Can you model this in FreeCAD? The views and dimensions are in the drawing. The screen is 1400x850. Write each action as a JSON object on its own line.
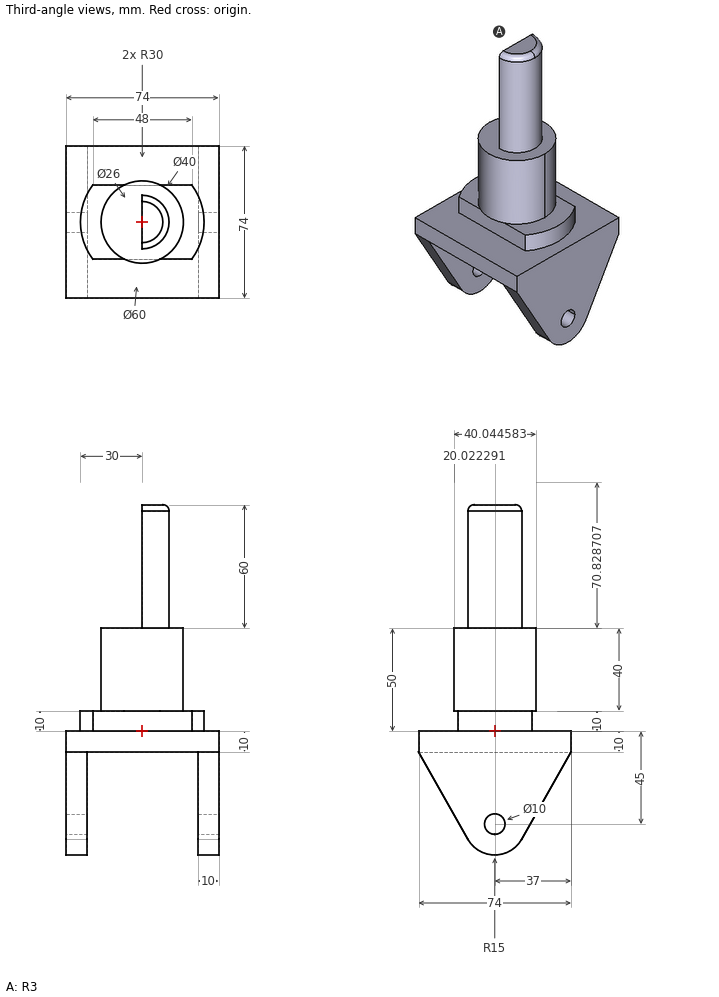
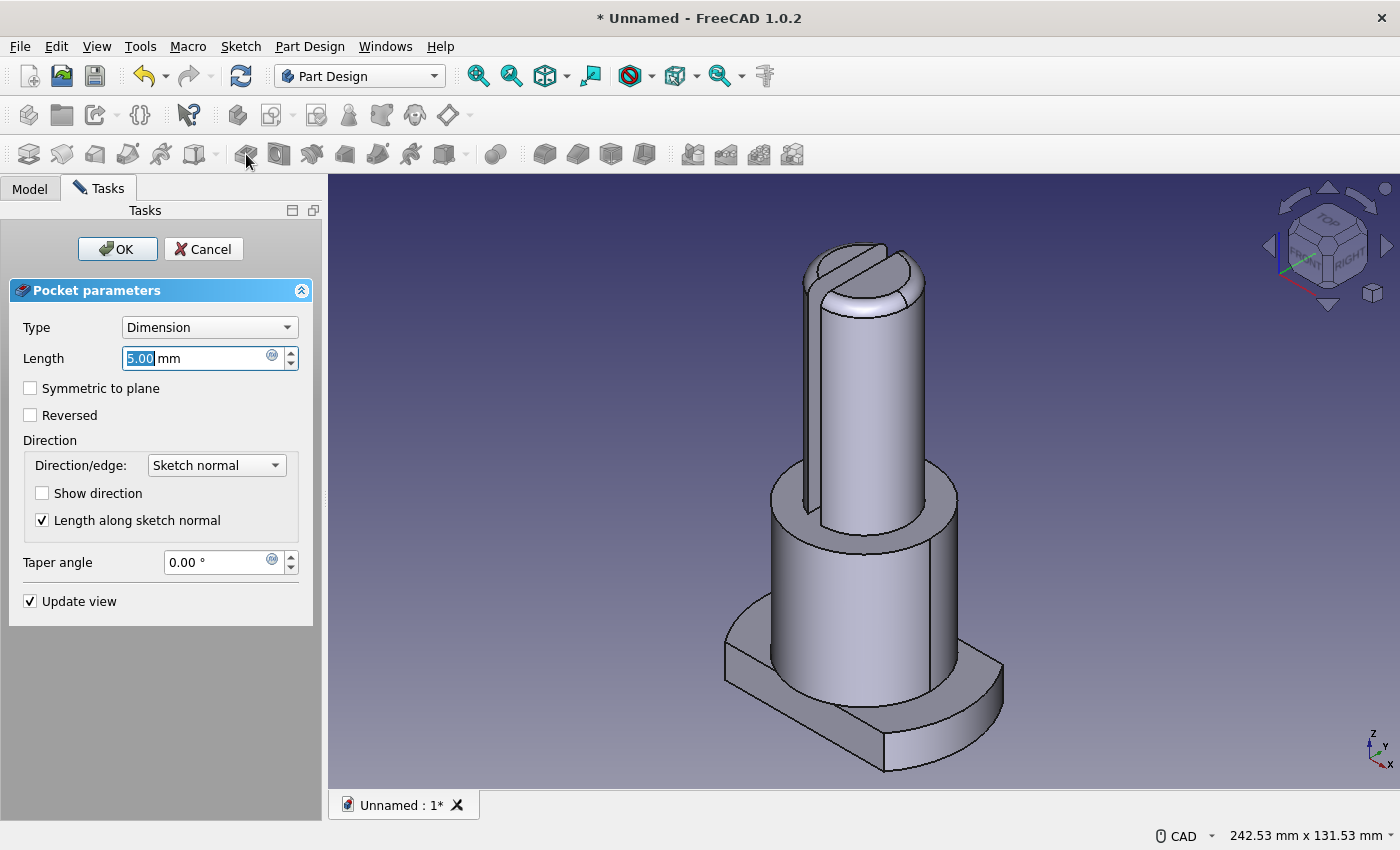
{"action": "type", "text": "30"}
{"action": "key", "text": "Tab"}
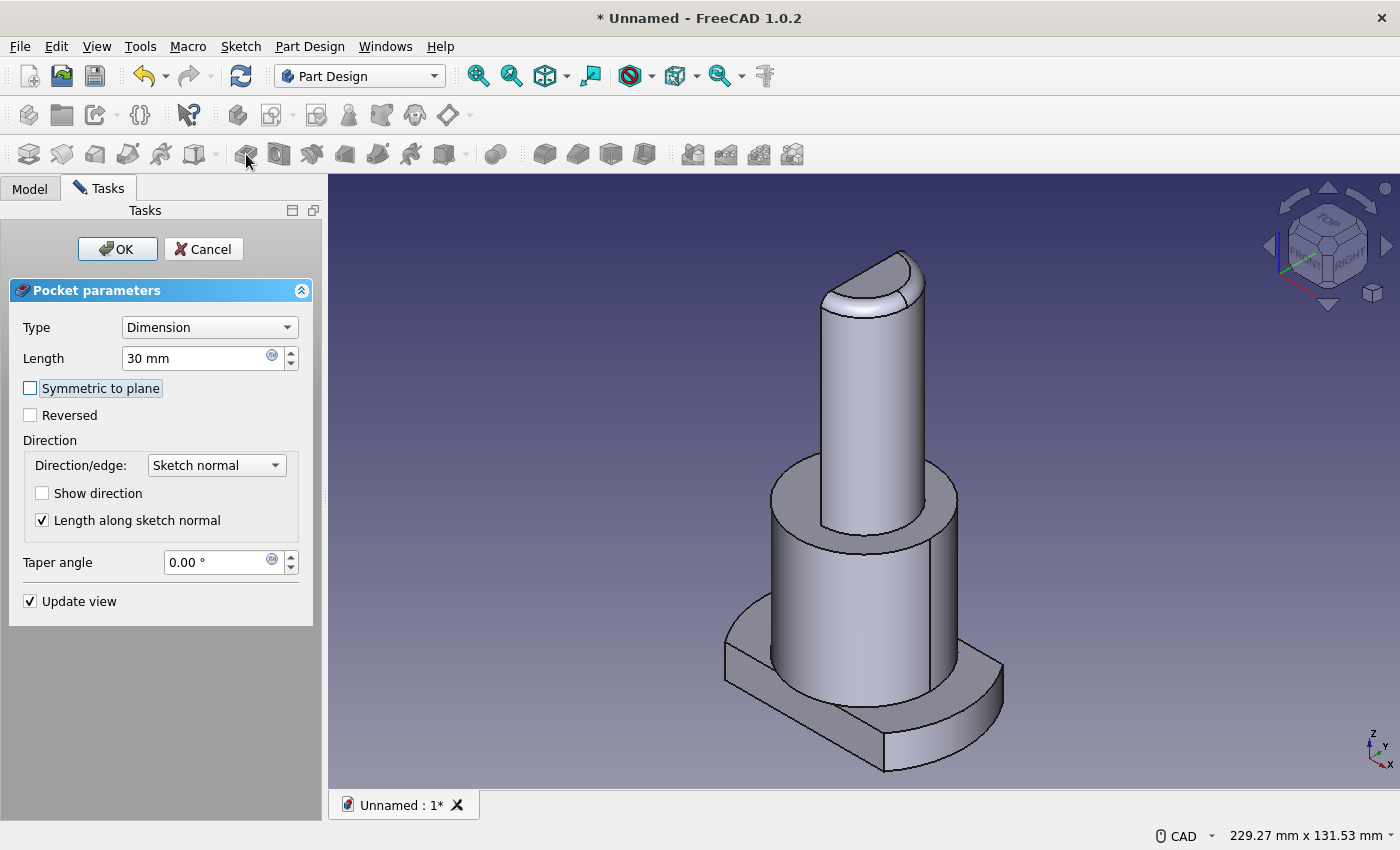
{"action": "left_click", "coordinate": [118, 249]}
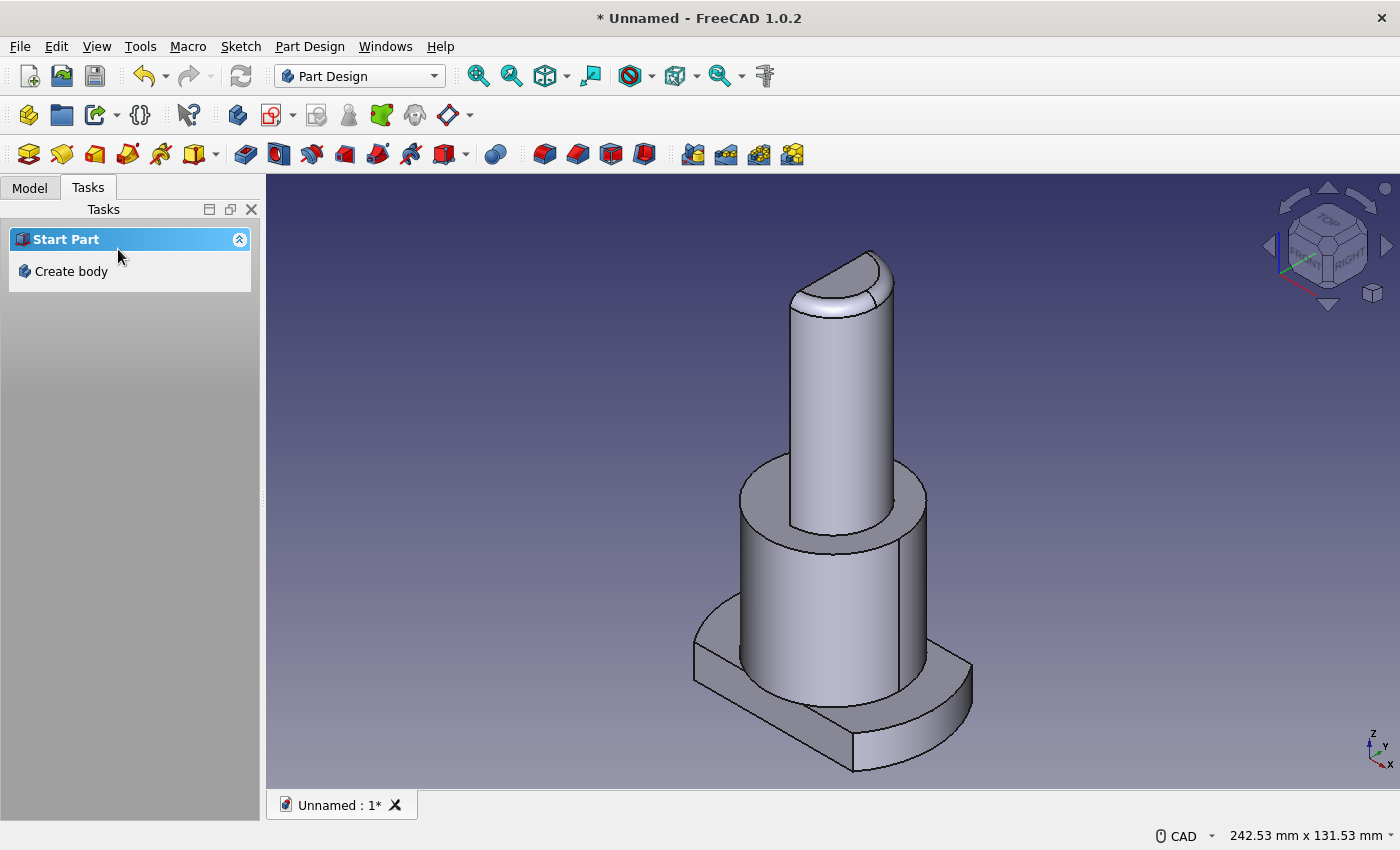
{"action": "key", "text": "5"}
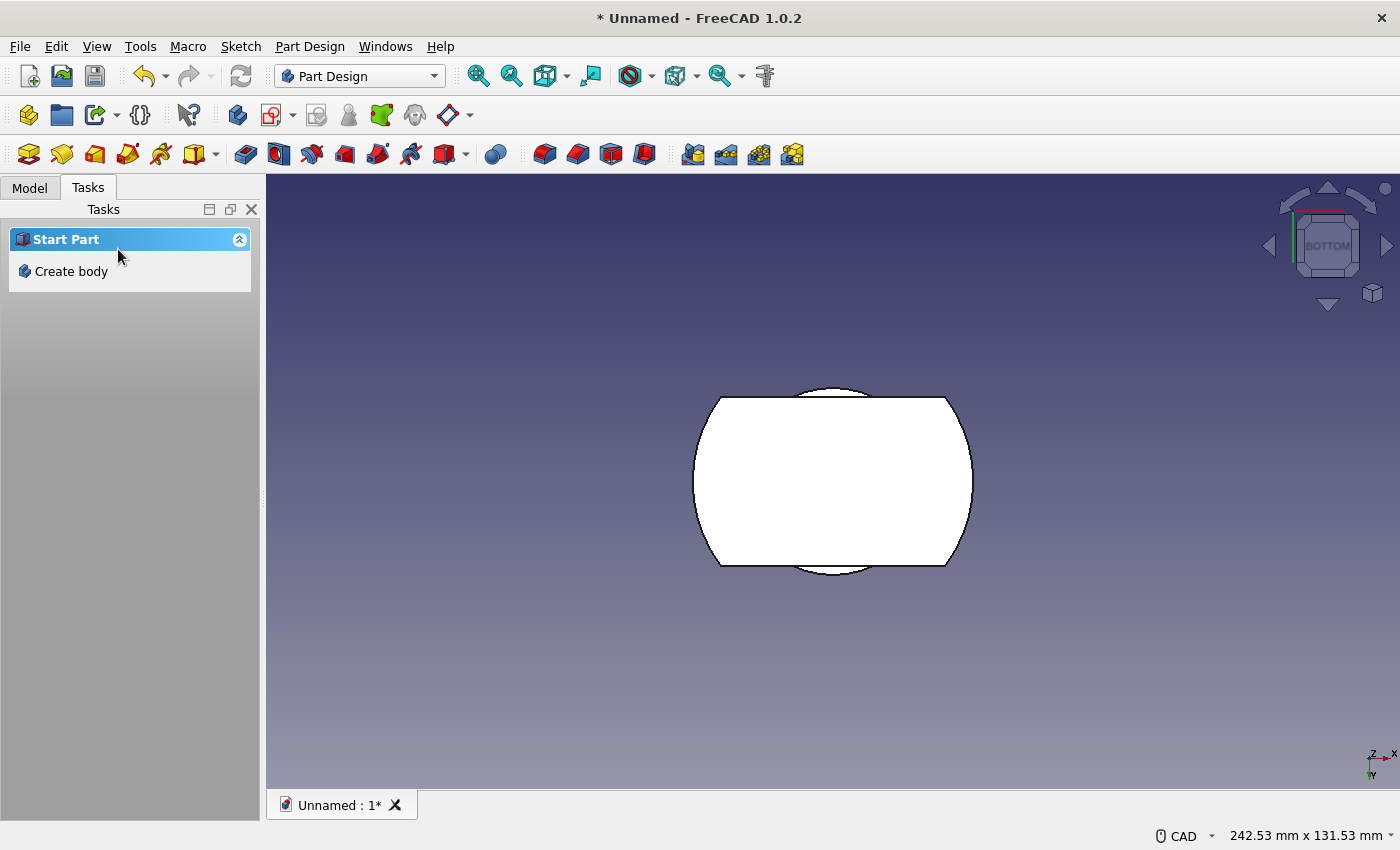
{"action": "left_click", "coordinate": [479, 76]}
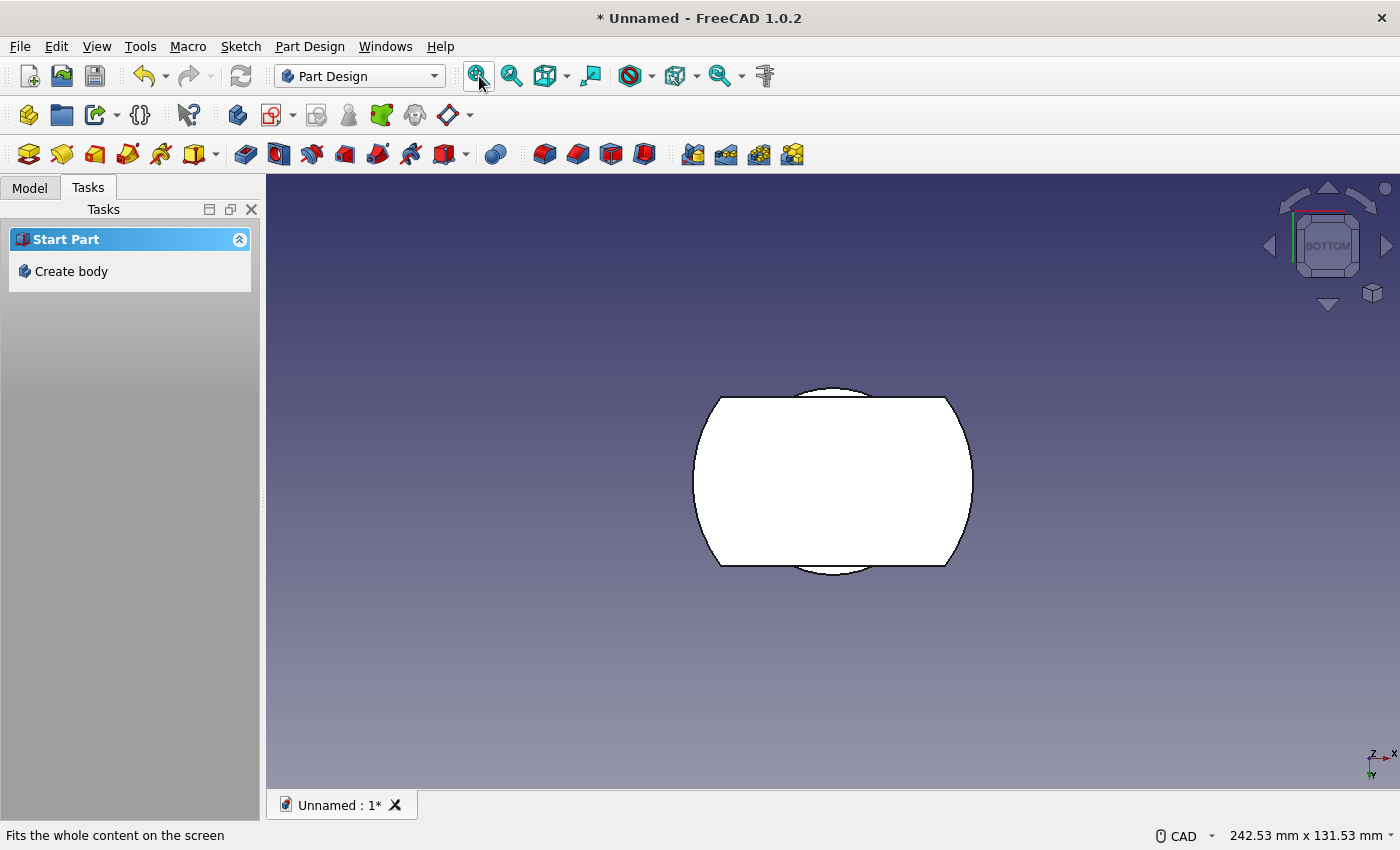
{"action": "left_click", "coordinate": [873, 480]}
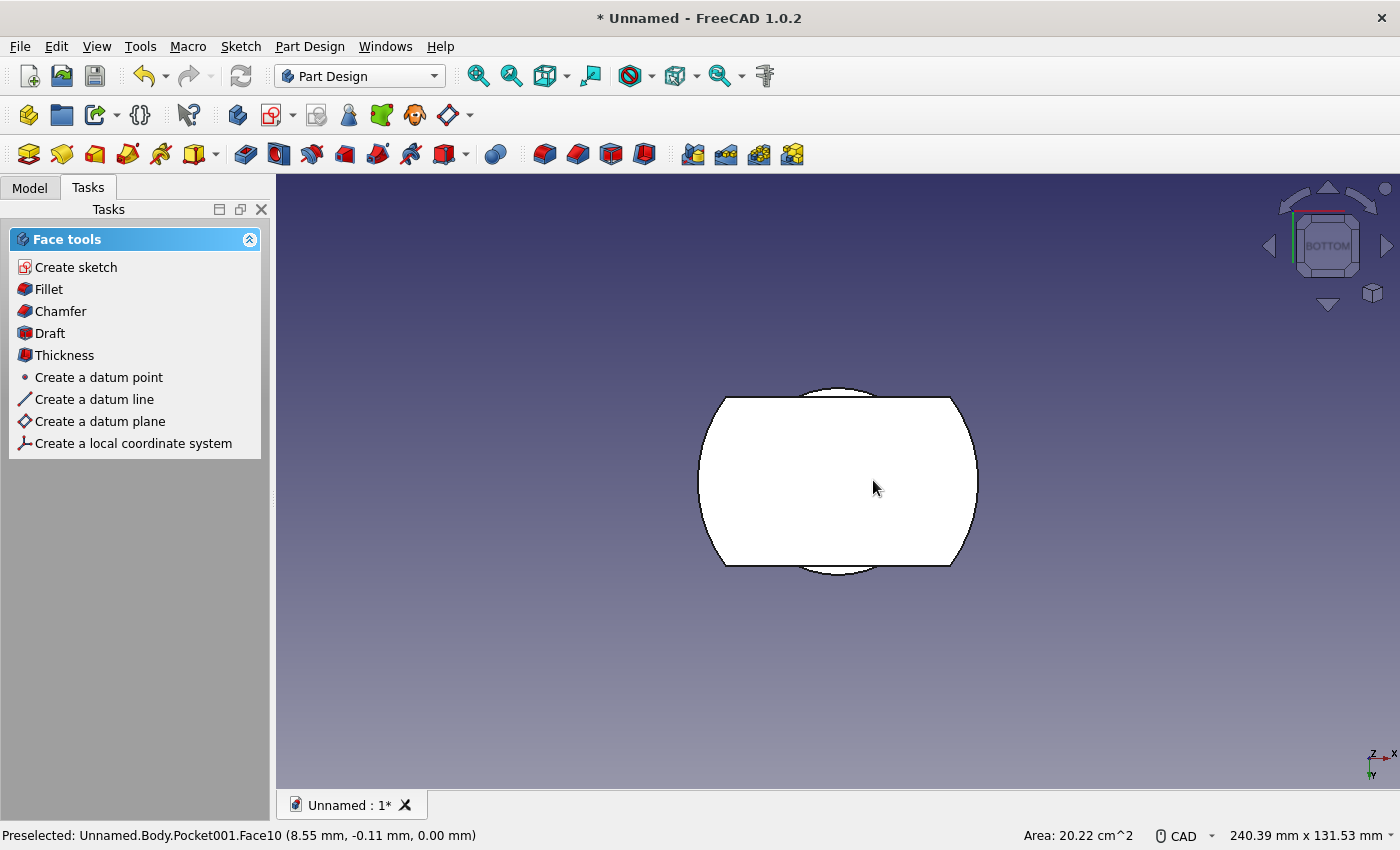
{"action": "left_click", "coordinate": [270, 116]}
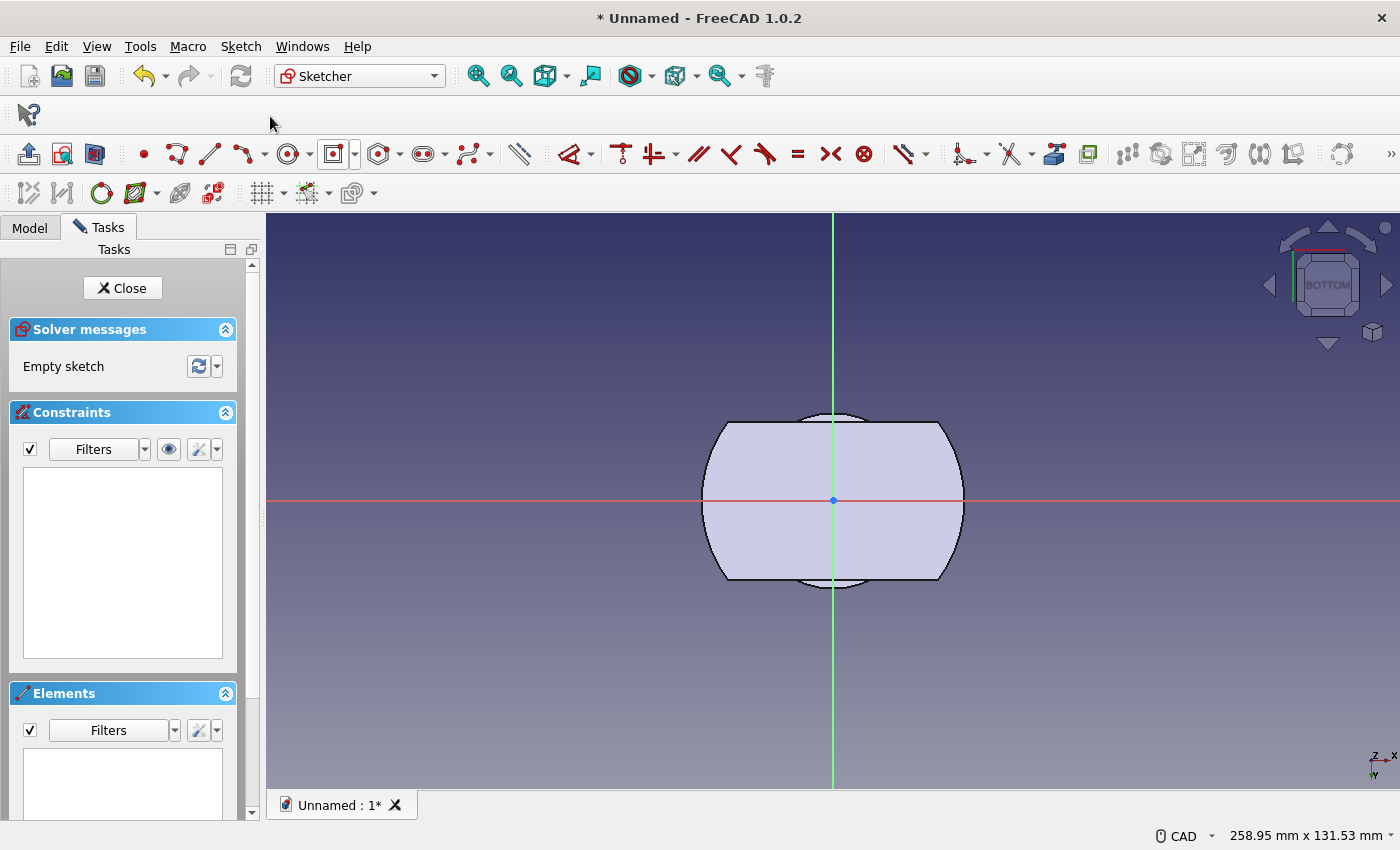
{"action": "key", "text": "g v"}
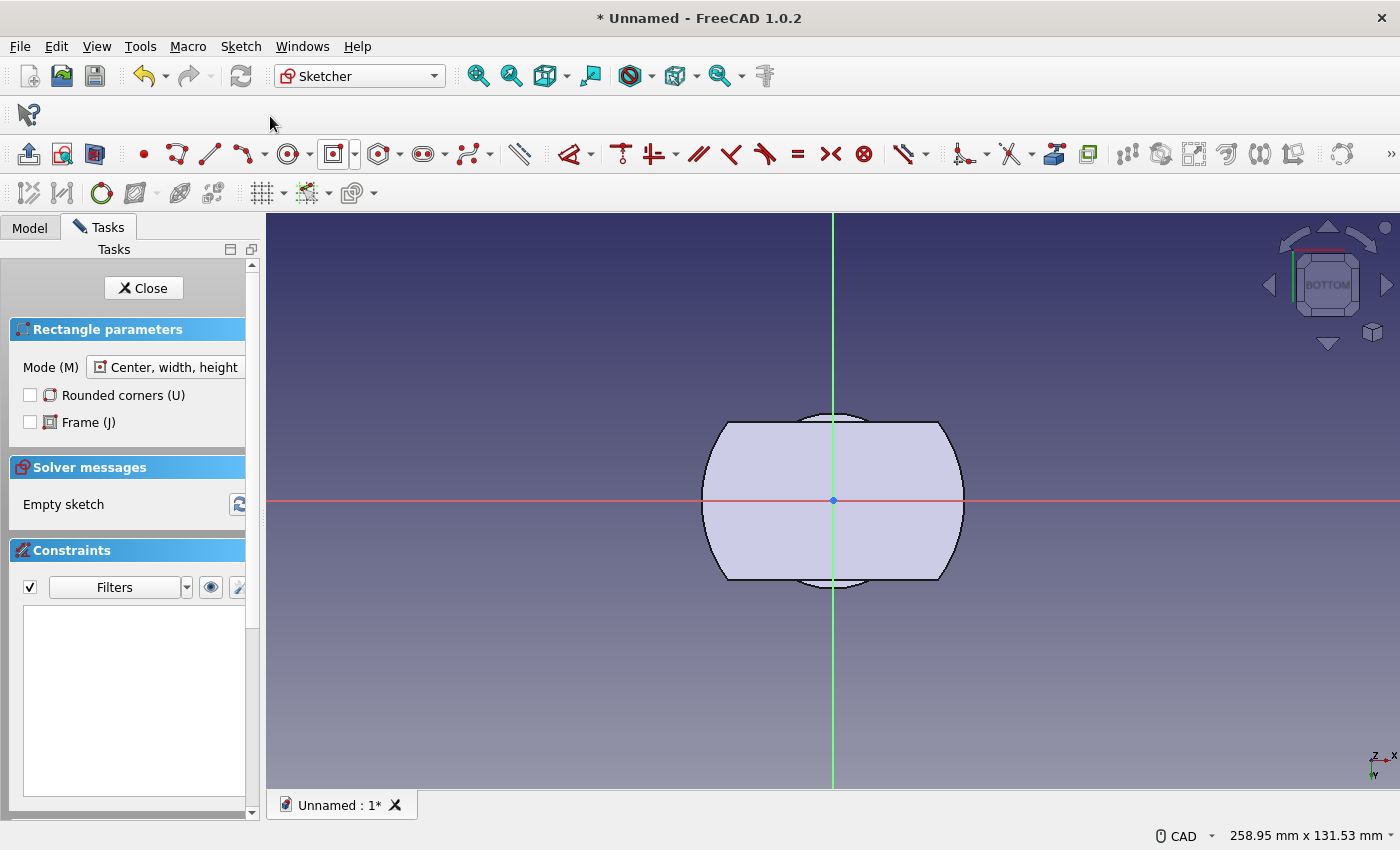
{"action": "left_click", "coordinate": [833, 501]}
{"action": "mouse_move", "coordinate": [995, 339]}